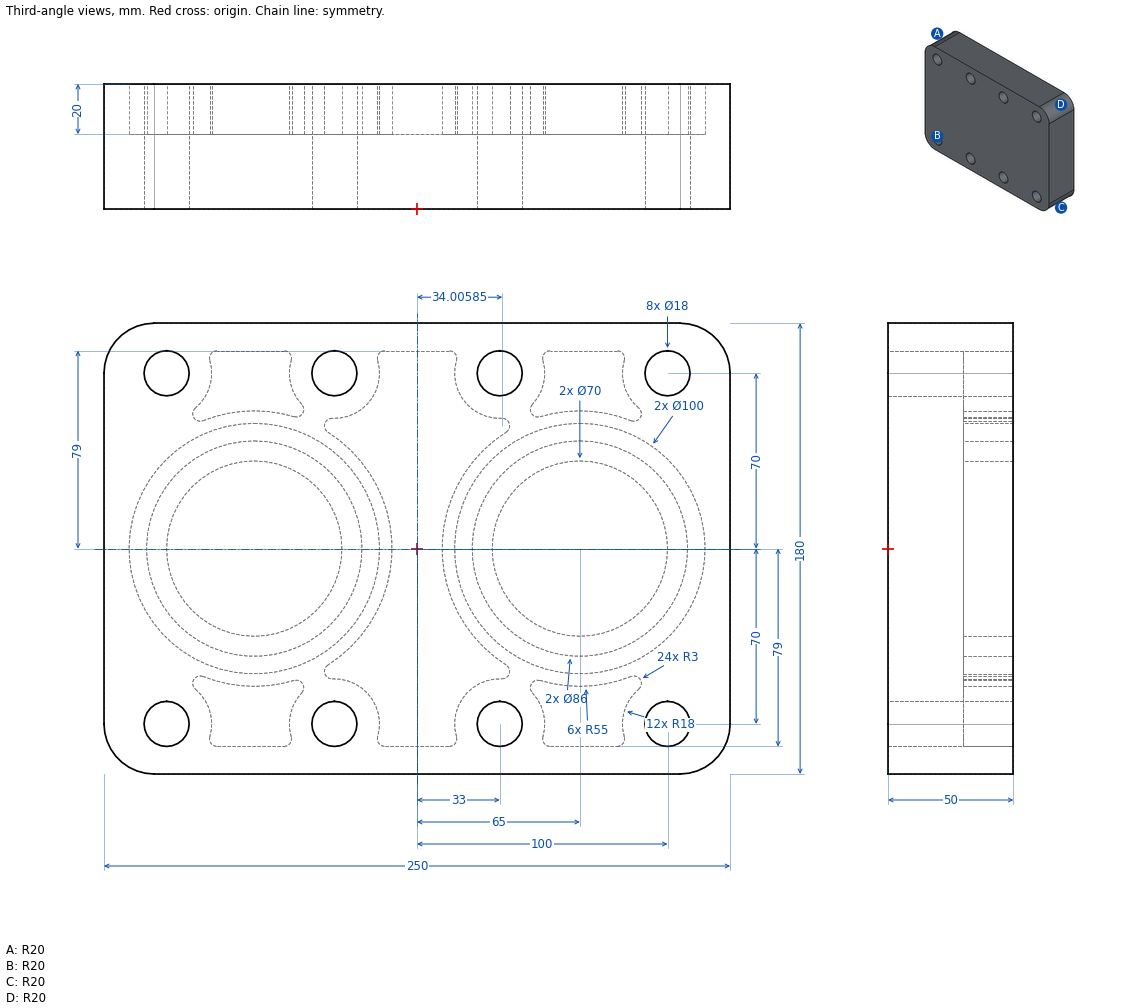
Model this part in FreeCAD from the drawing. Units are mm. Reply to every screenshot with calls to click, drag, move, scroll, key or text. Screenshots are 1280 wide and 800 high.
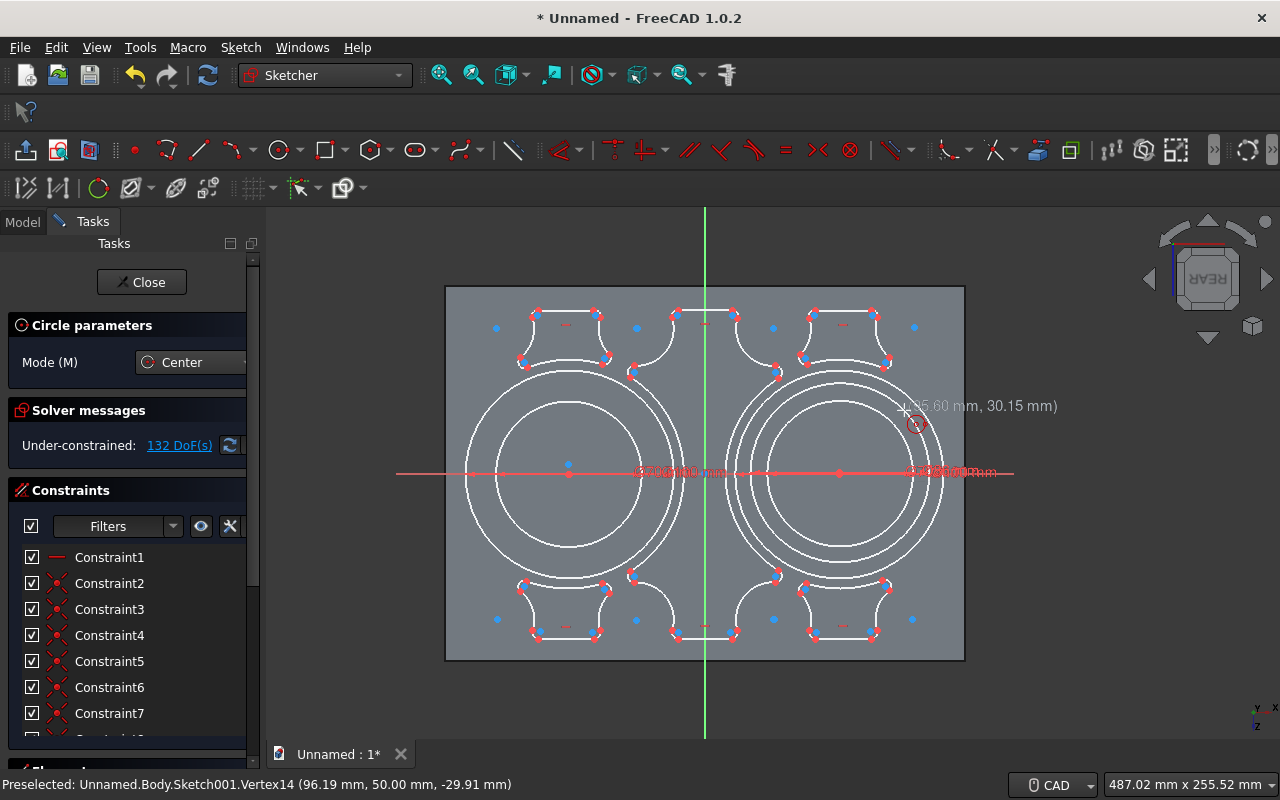
click(570, 474)
move(633, 410)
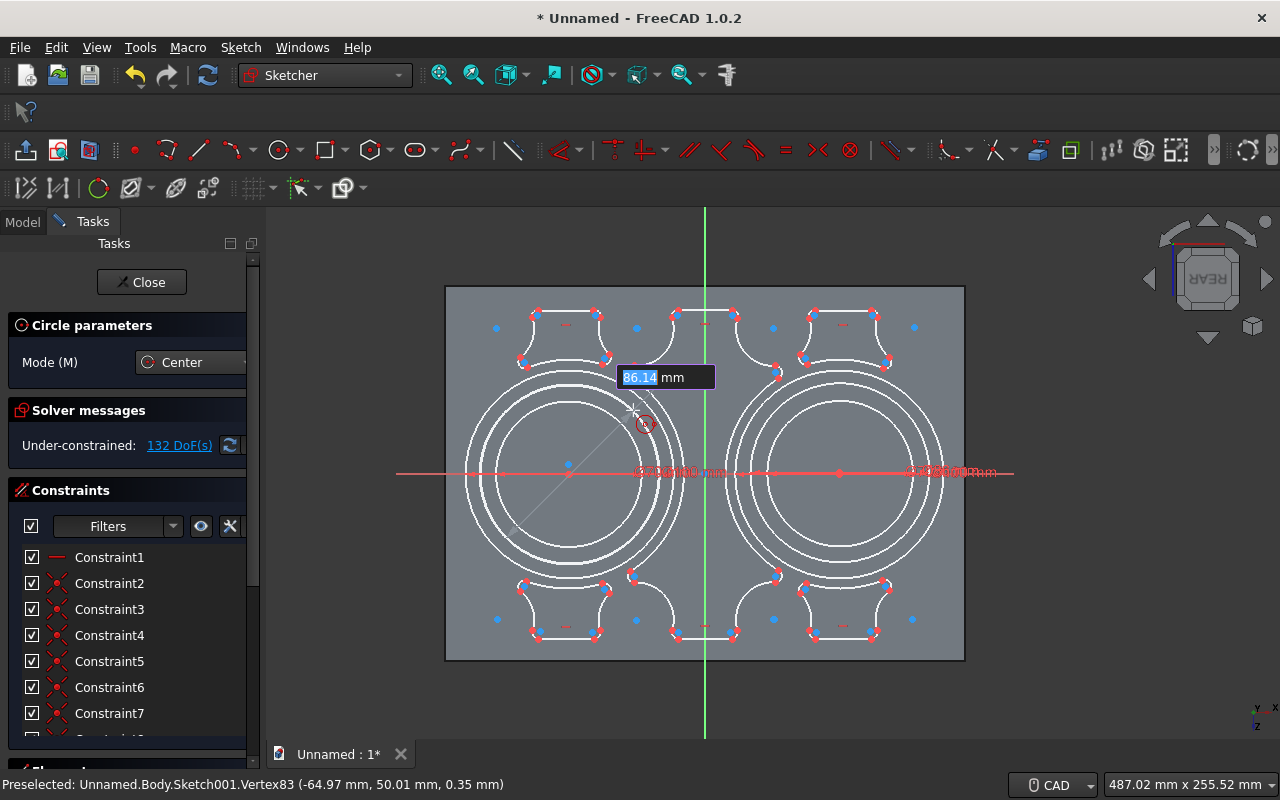
text(86)
key(Return)
key(Escape)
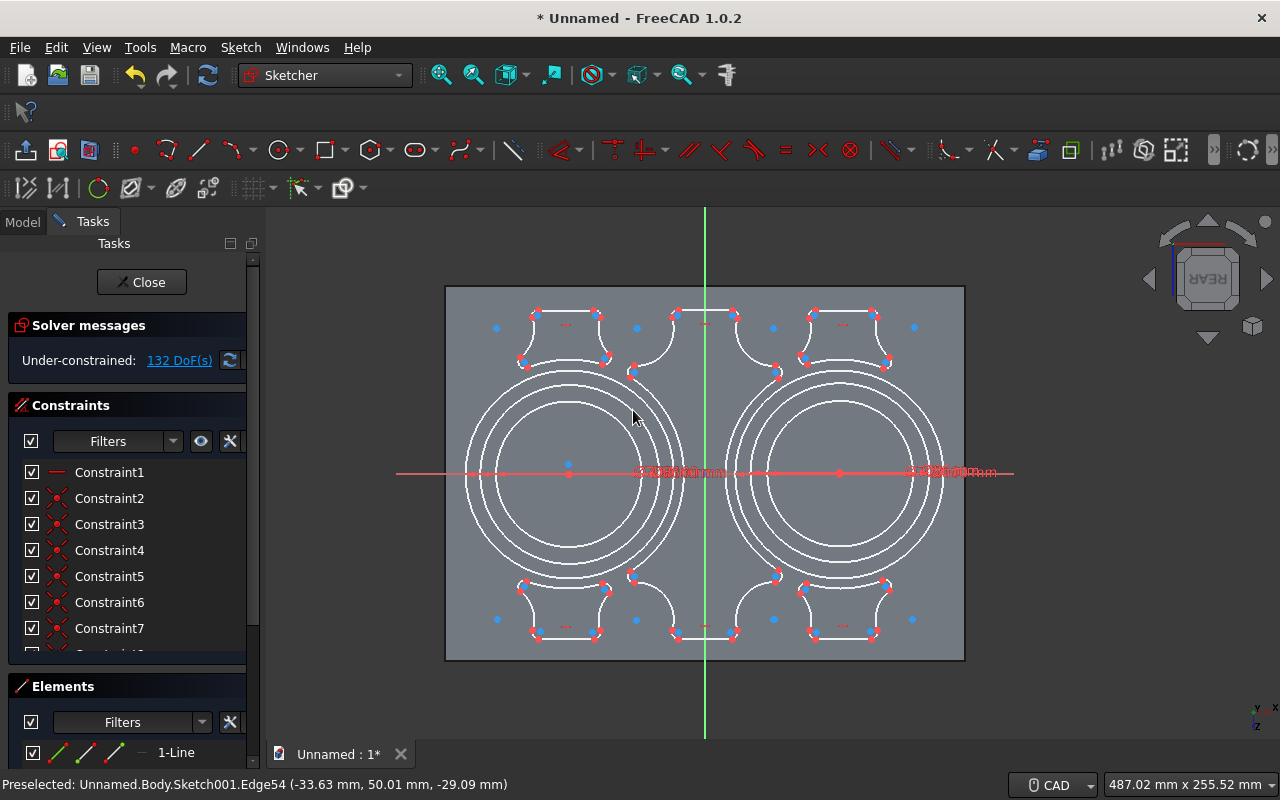
click(855, 311)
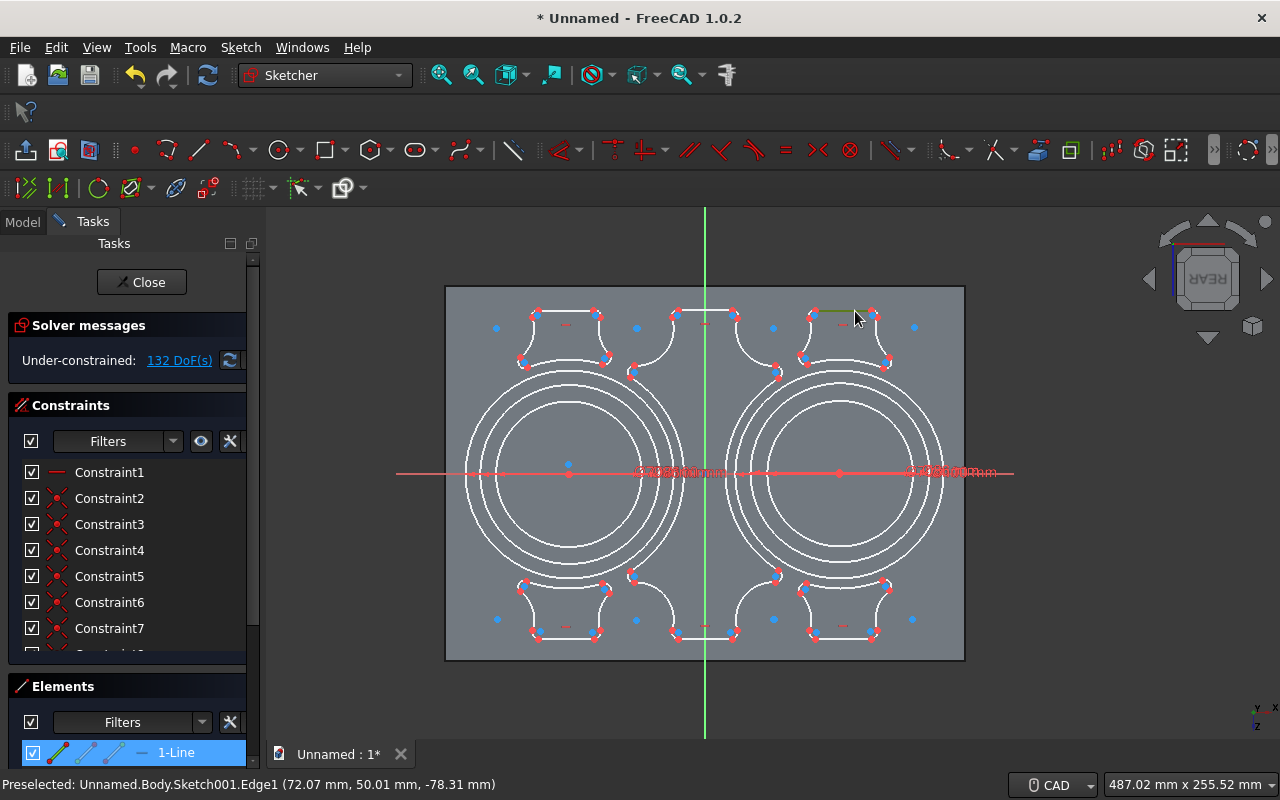
scroll(810, 312, up, 5)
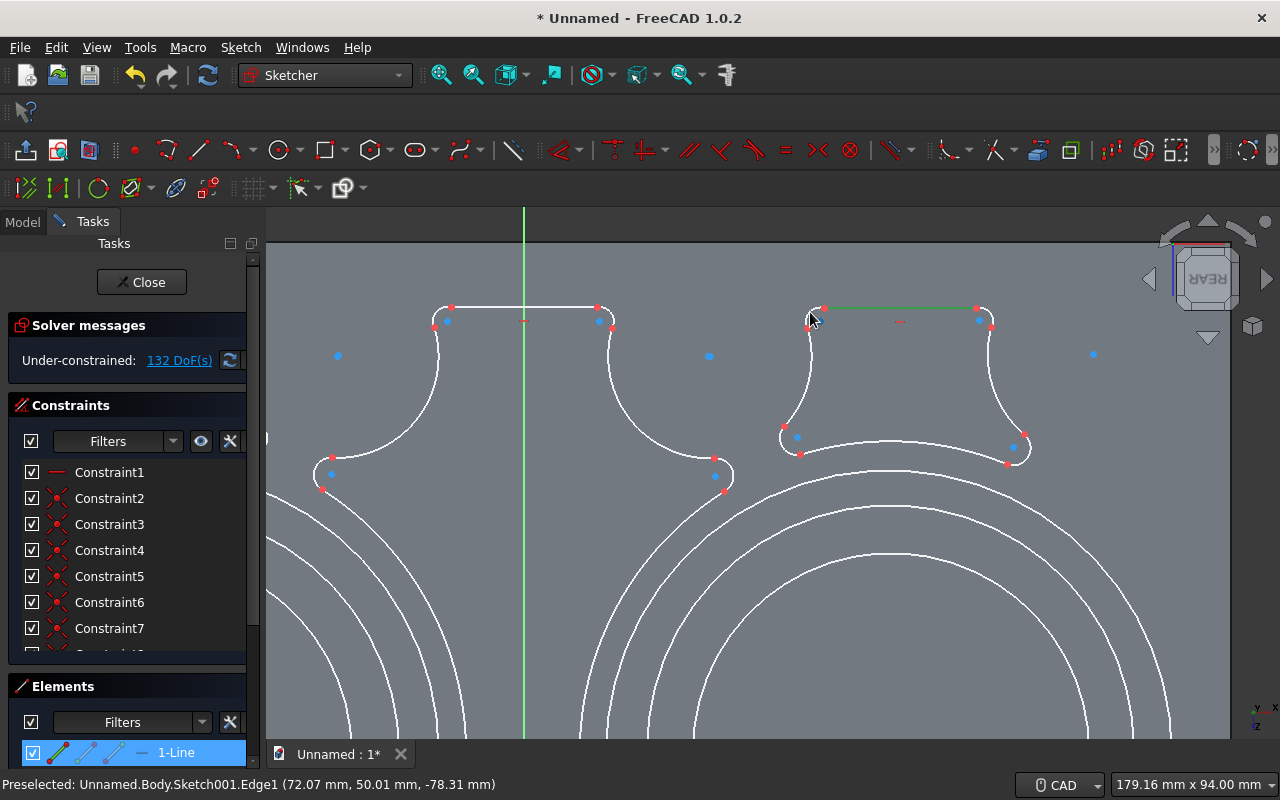
click(809, 312)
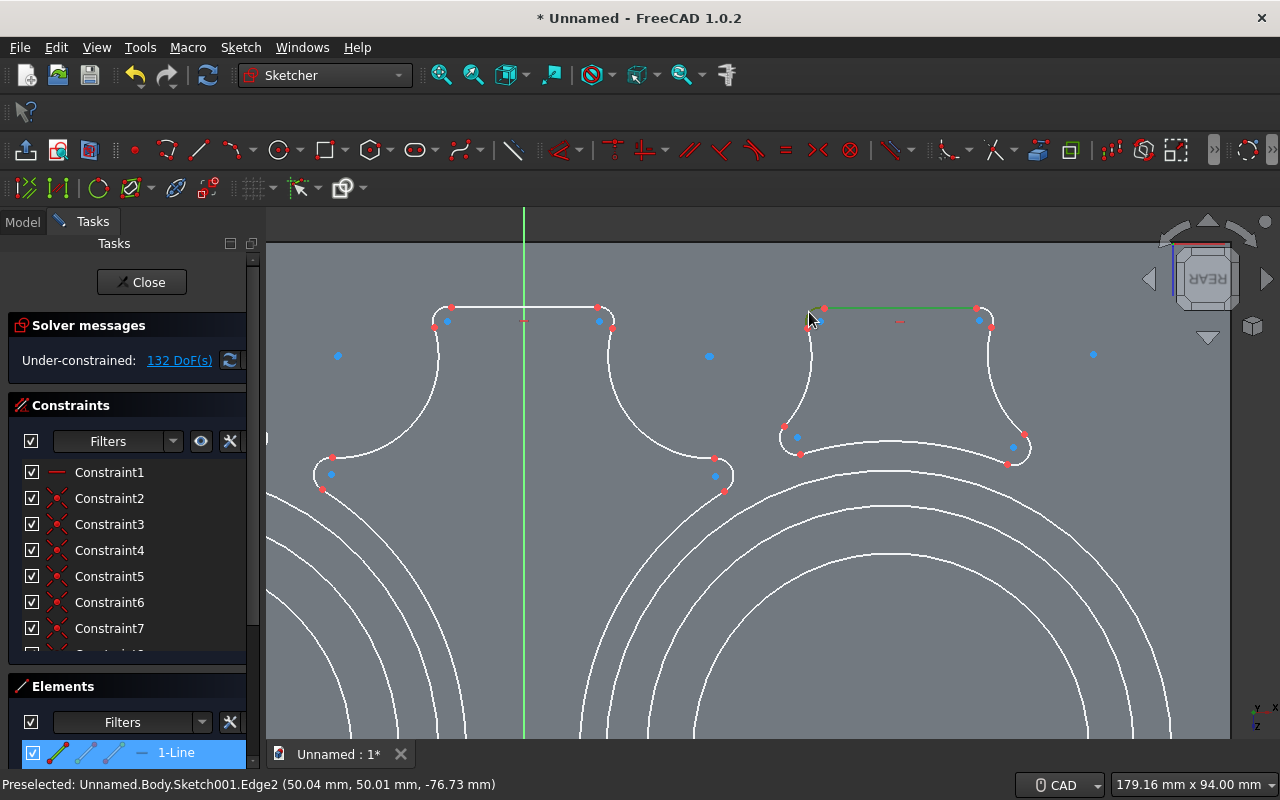
click(754, 150)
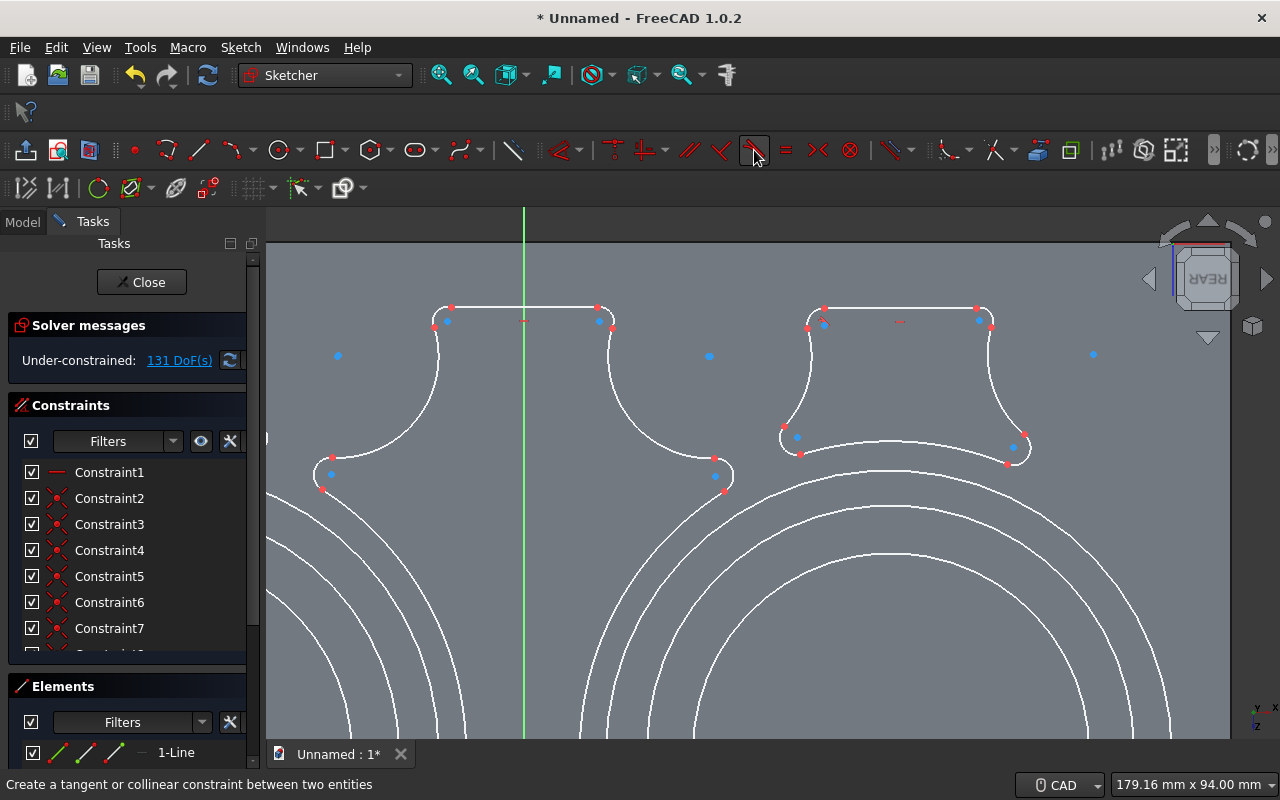
click(931, 308)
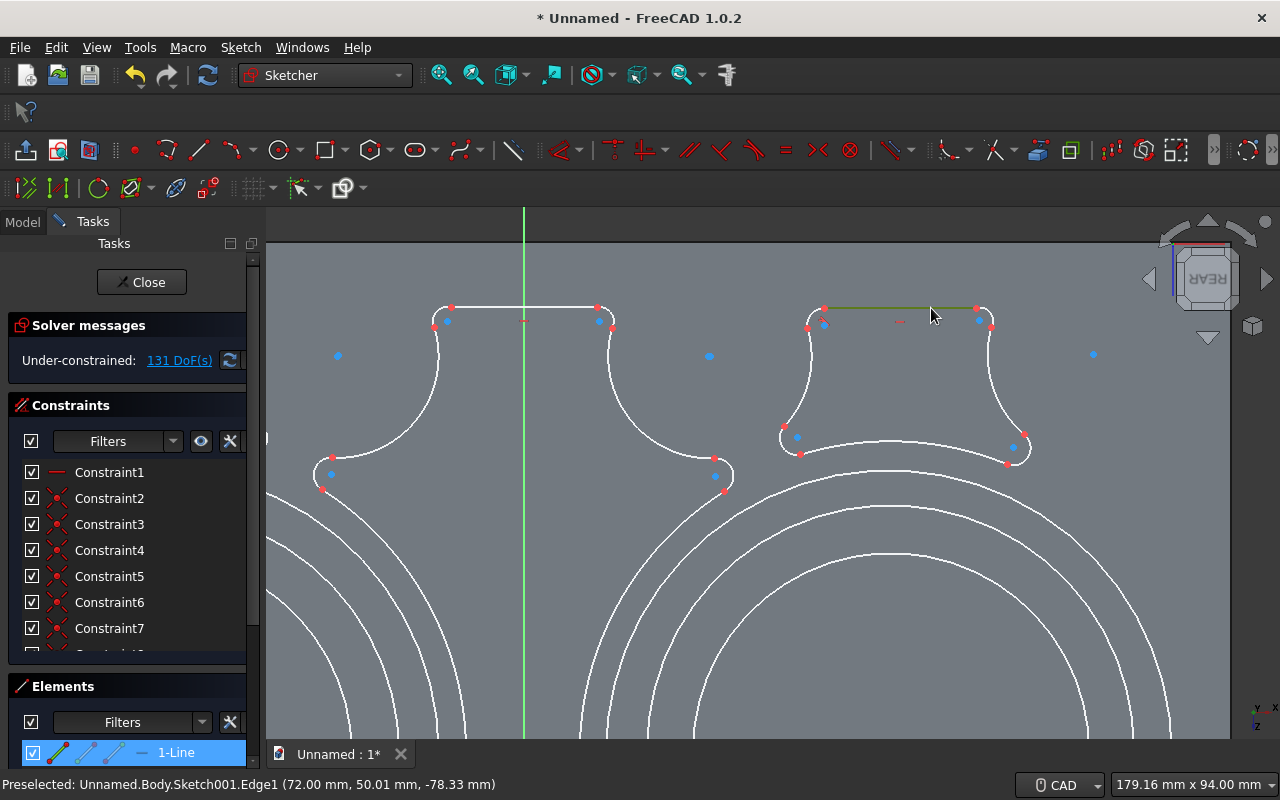
click(990, 313)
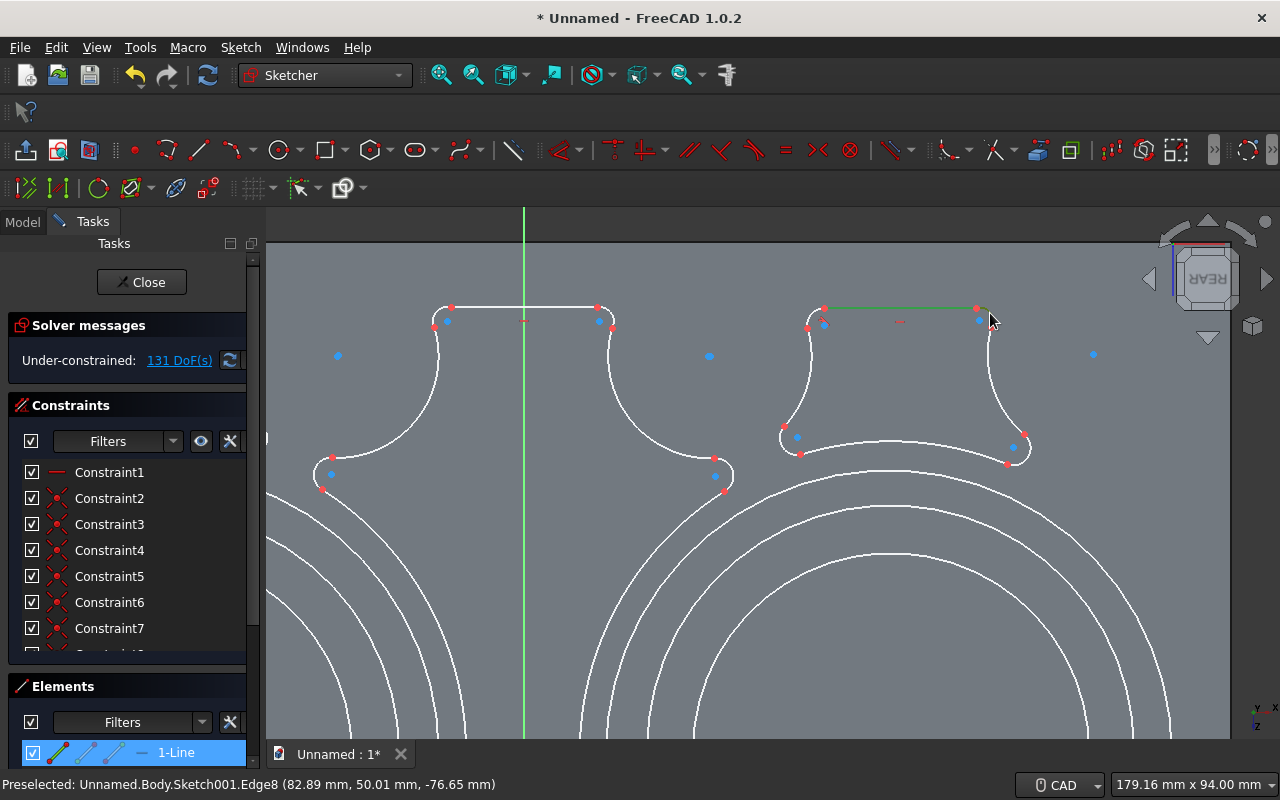
click(754, 150)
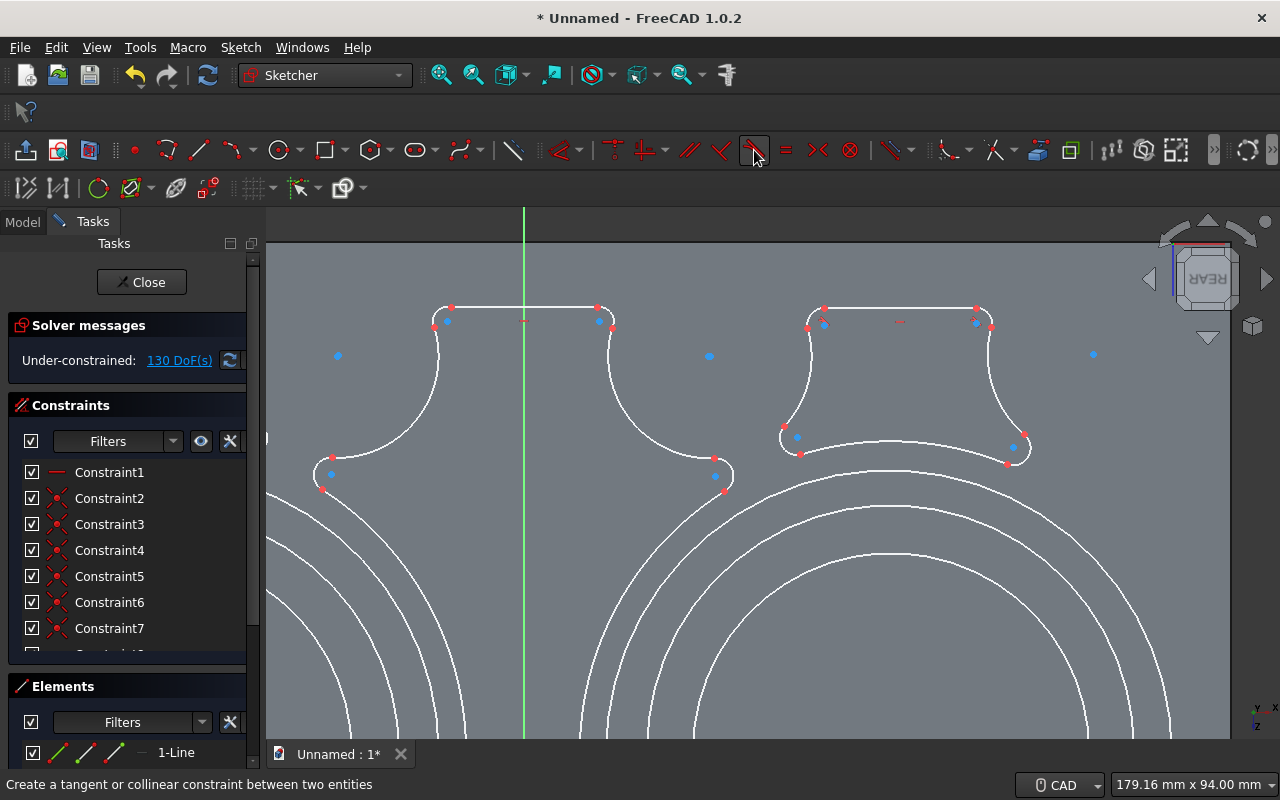
click(811, 314)